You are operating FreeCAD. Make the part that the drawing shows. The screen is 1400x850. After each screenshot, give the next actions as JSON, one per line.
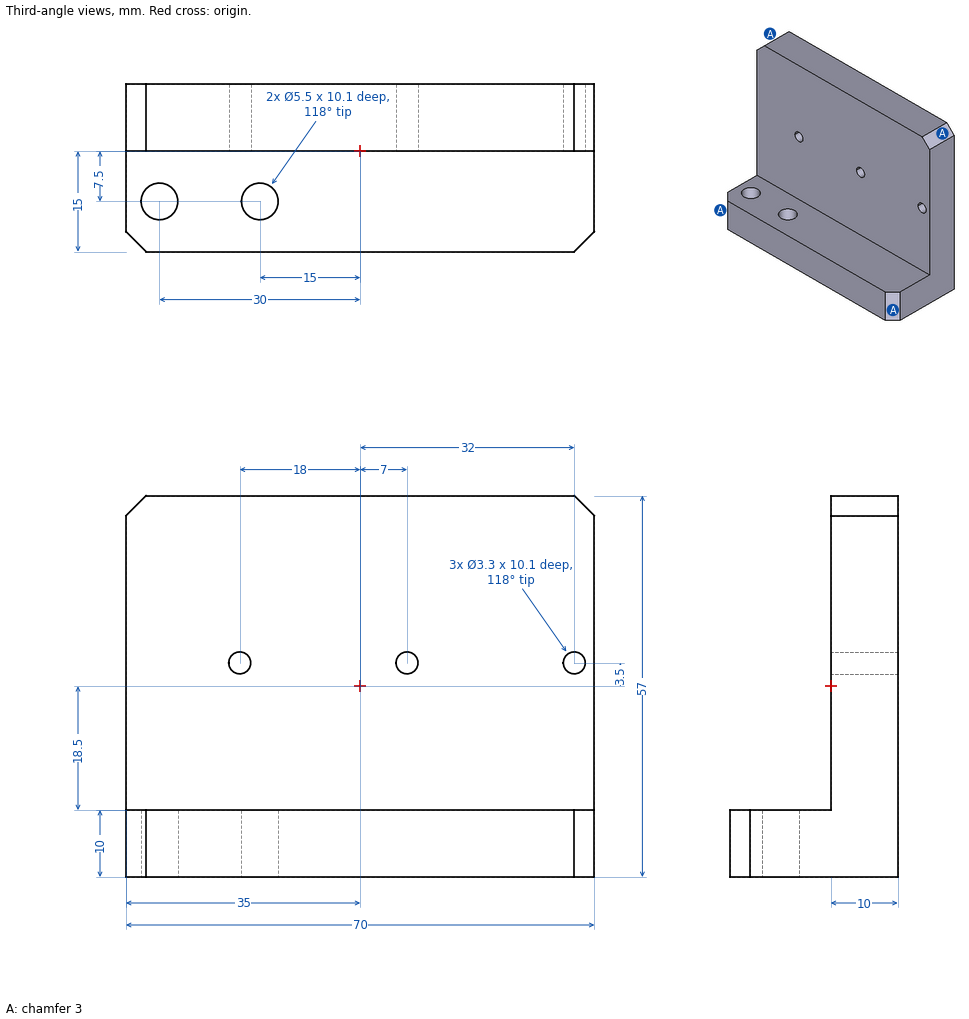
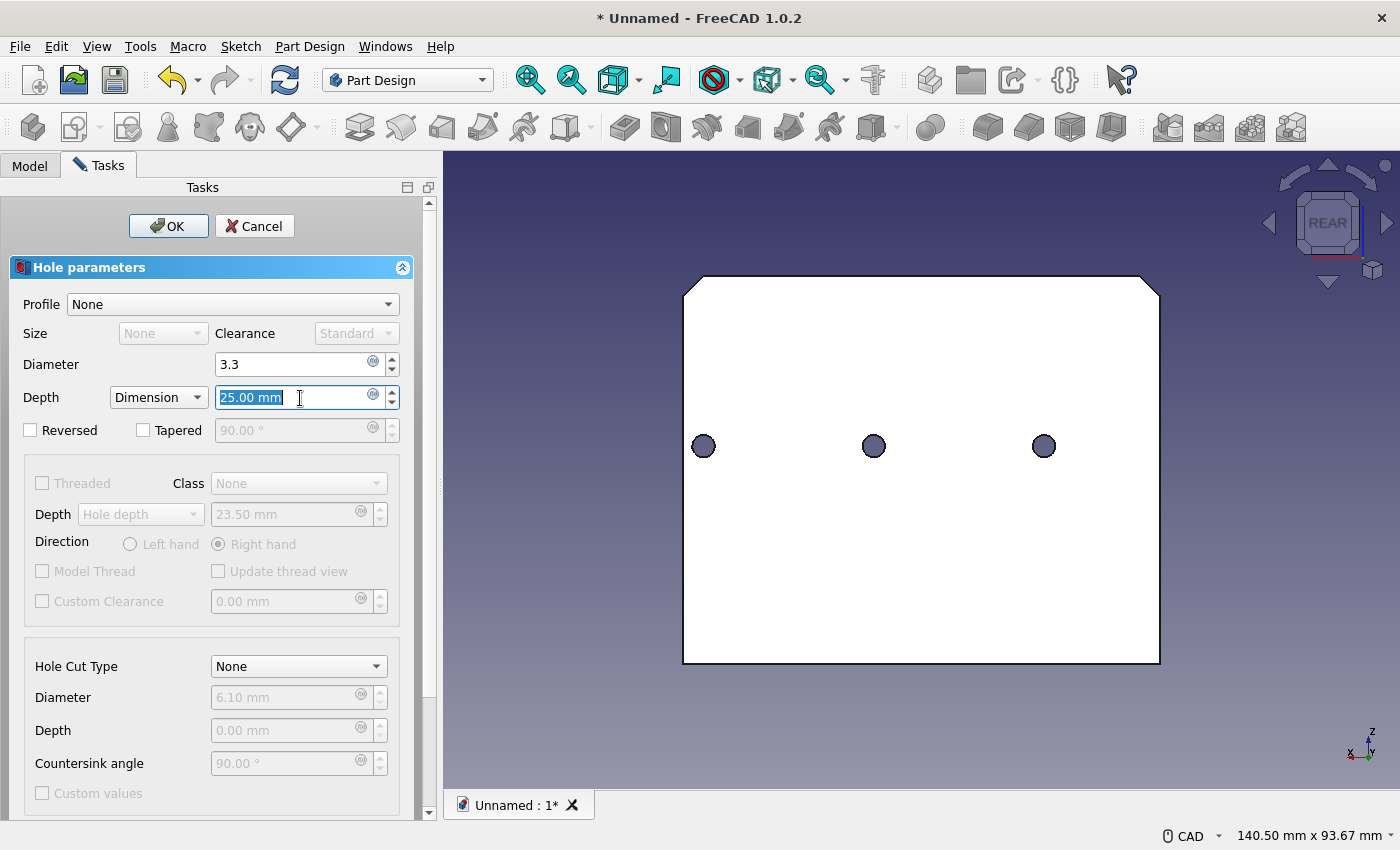
{"action": "type", "text": "10.1"}
{"action": "key", "text": "Tab"}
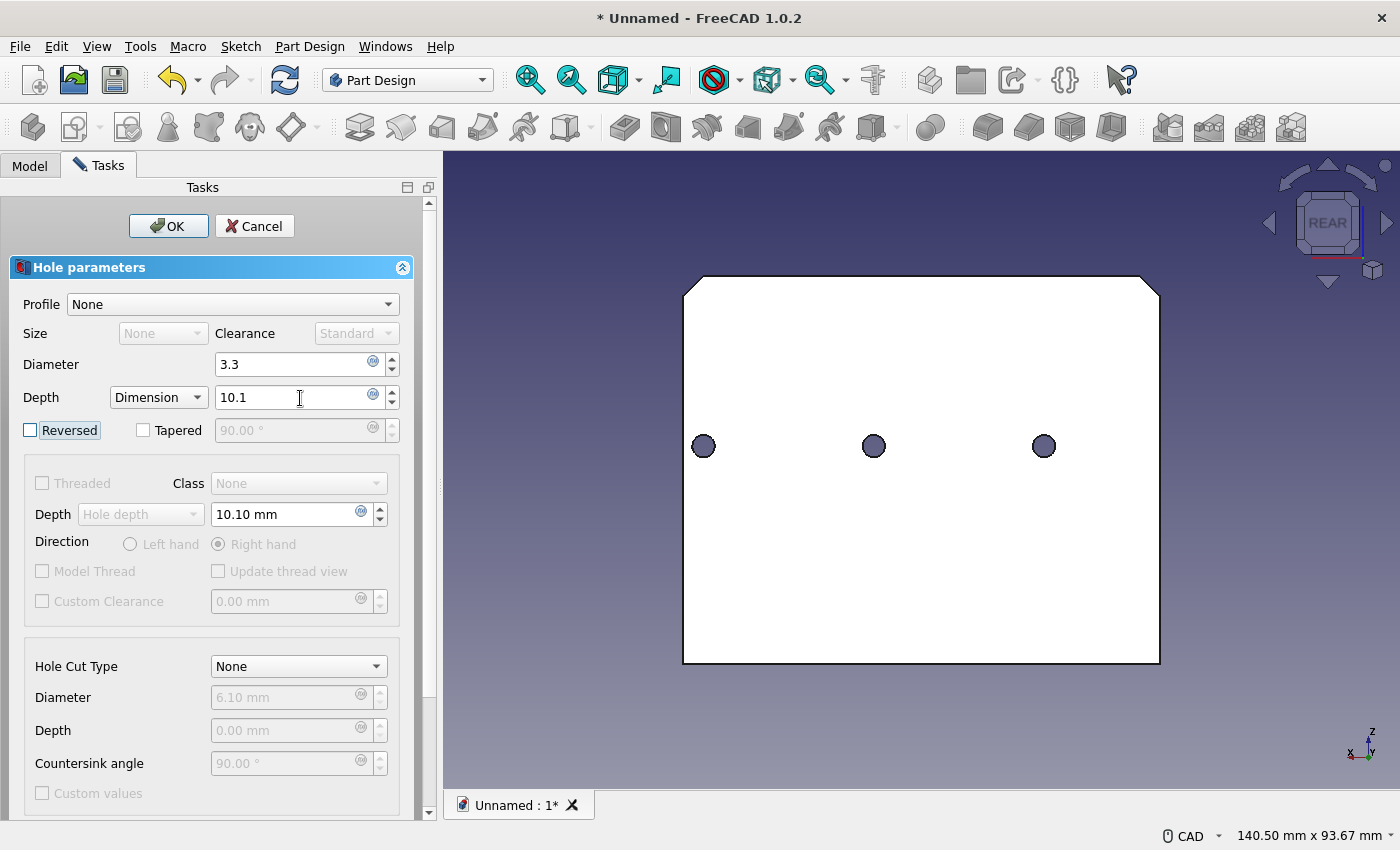
{"action": "left_click", "coordinate": [169, 226]}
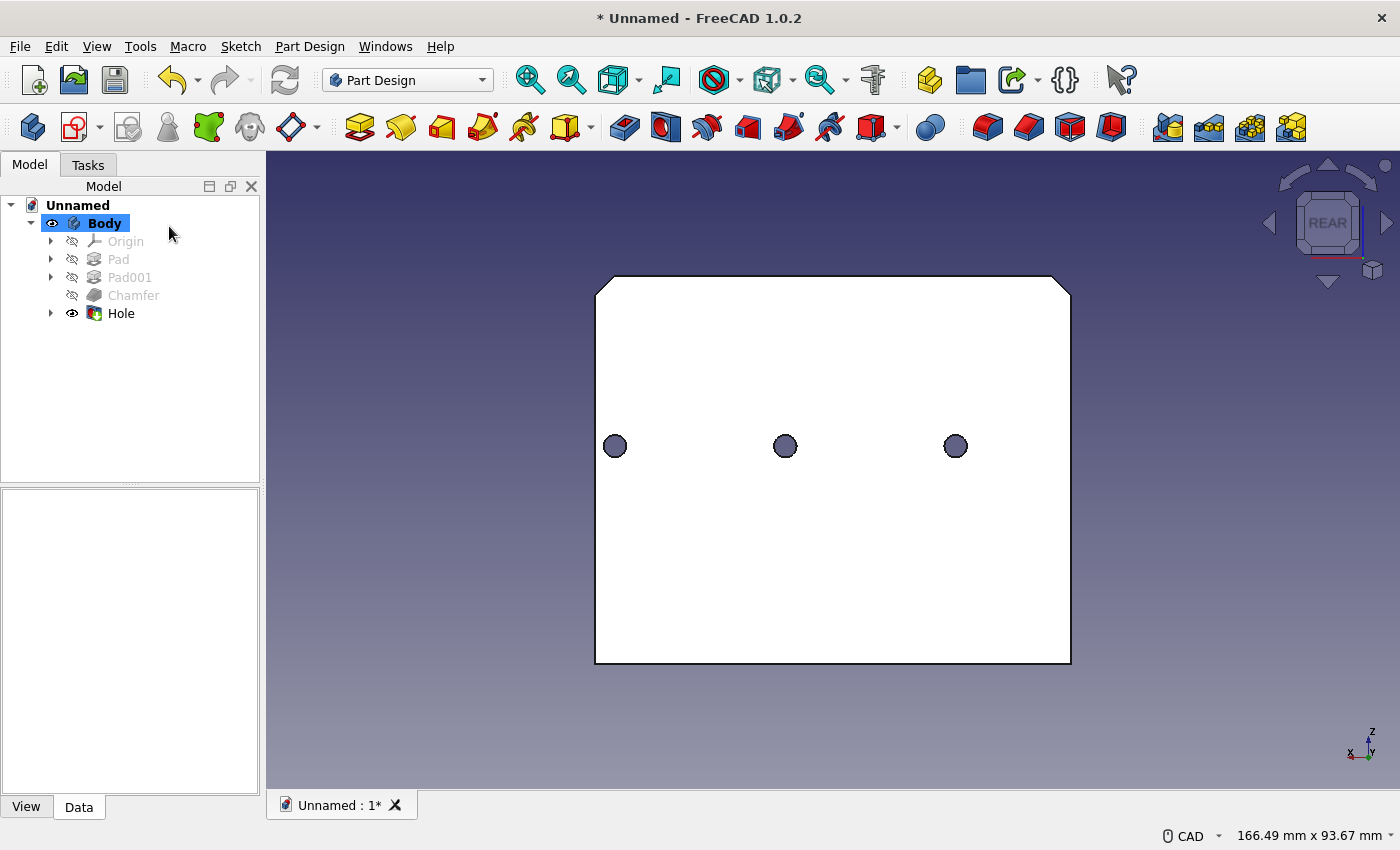
{"action": "key", "text": "0"}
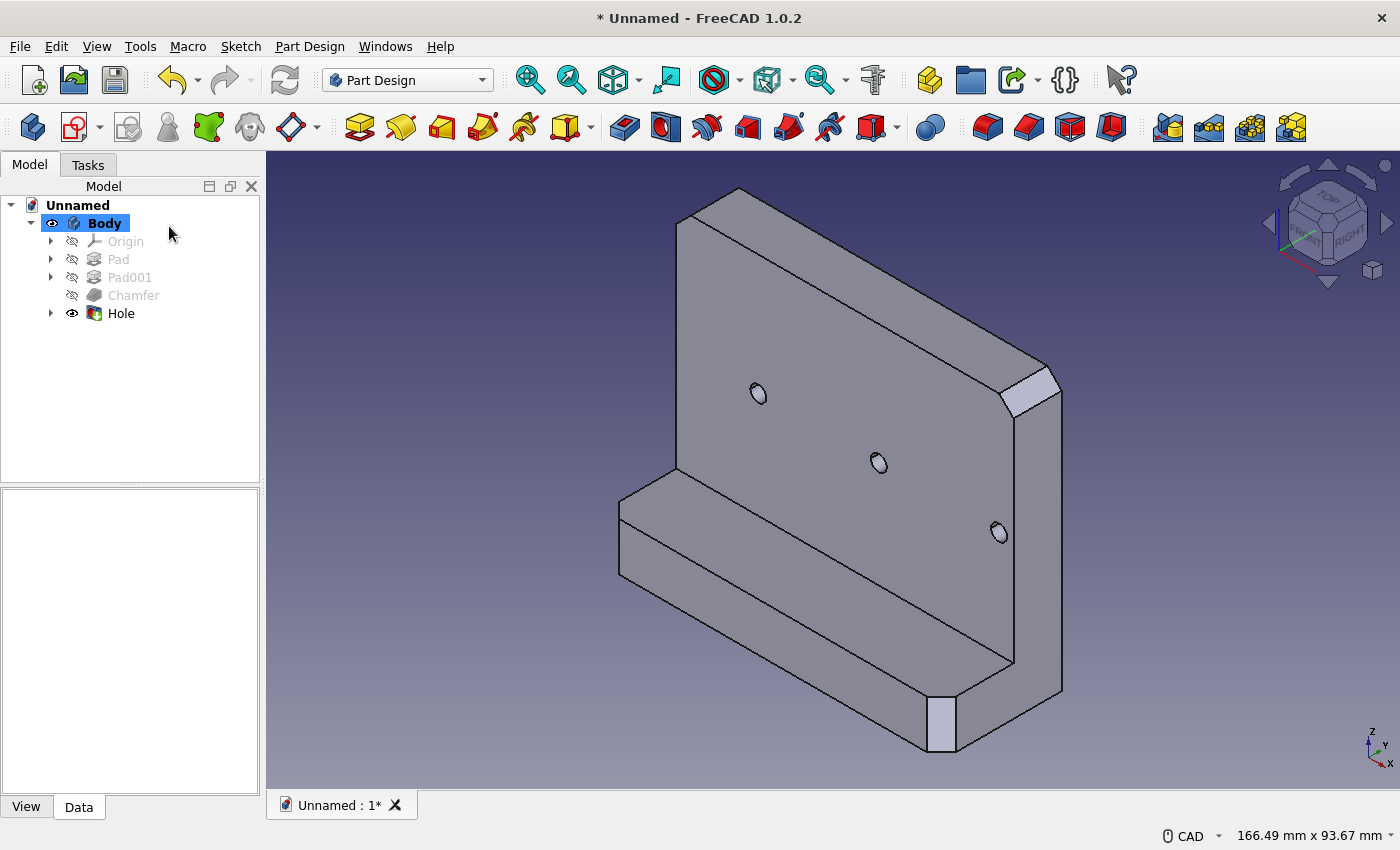
{"action": "left_click", "coordinate": [905, 641]}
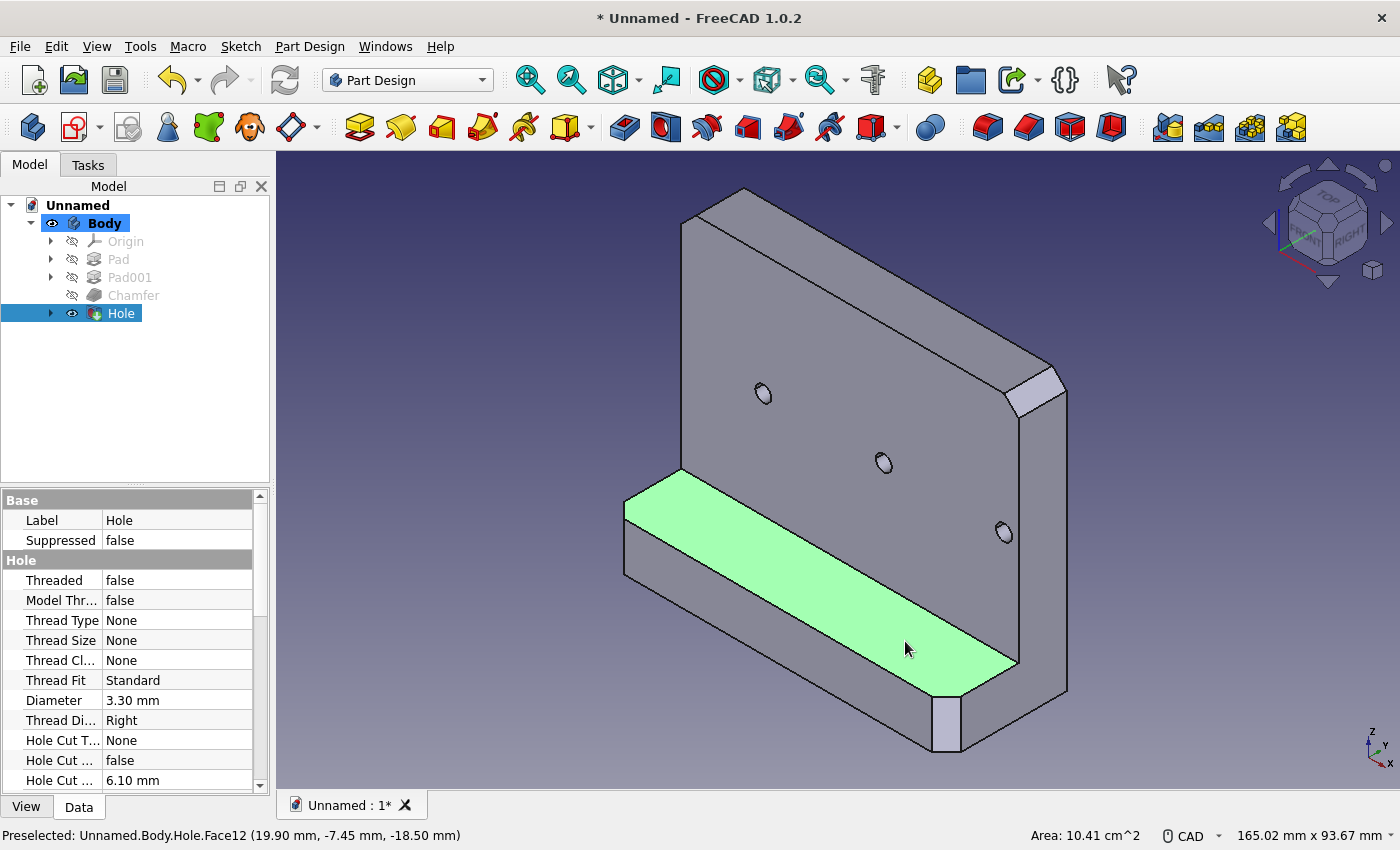
{"action": "left_click", "coordinate": [74, 128]}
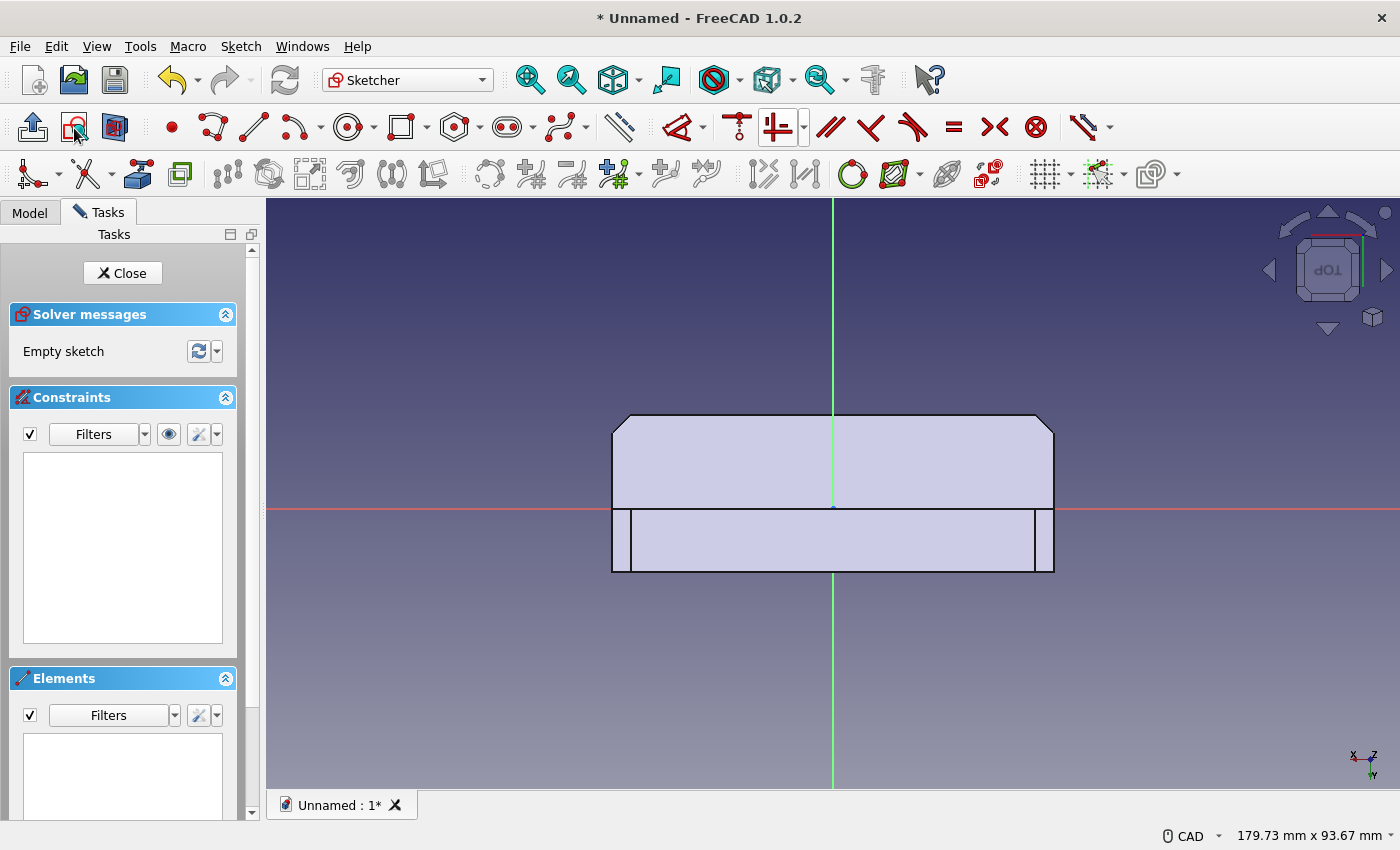
{"action": "scroll", "coordinate": [1010, 470], "scroll_direction": "up", "scroll_amount": 6}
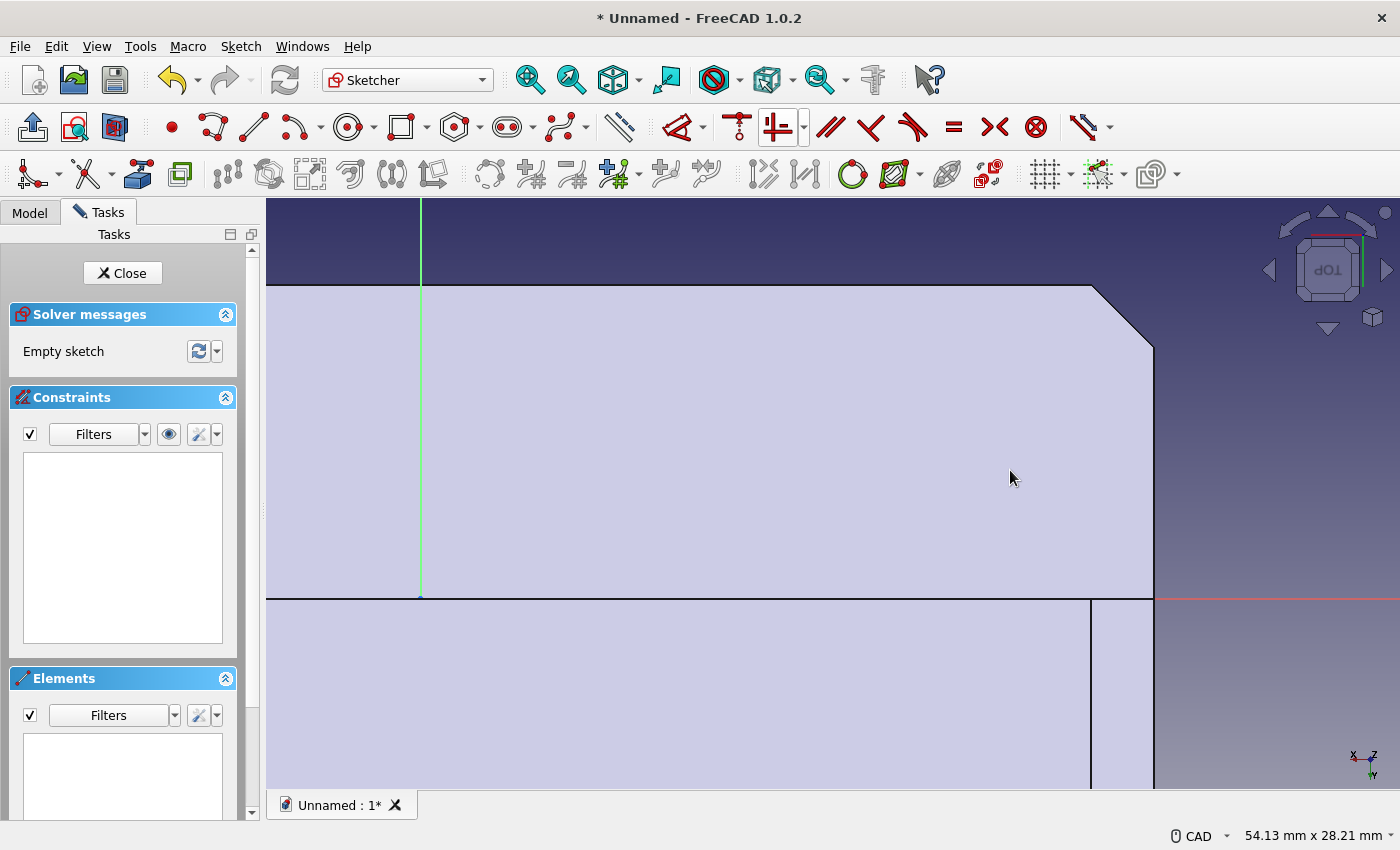
{"action": "left_click", "coordinate": [348, 128]}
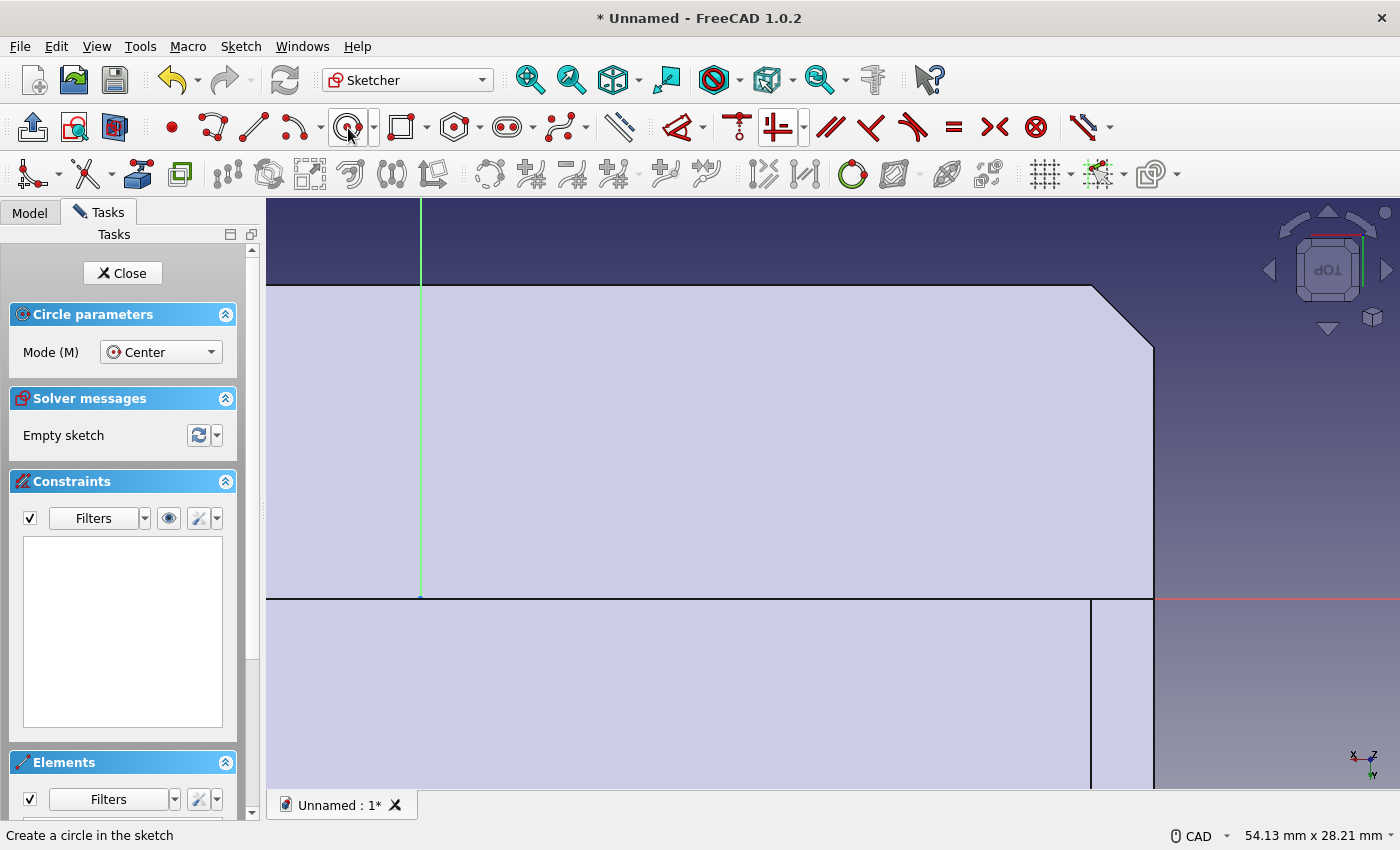
{"action": "left_click", "coordinate": [735, 442]}
{"action": "left_click", "coordinate": [776, 401]}